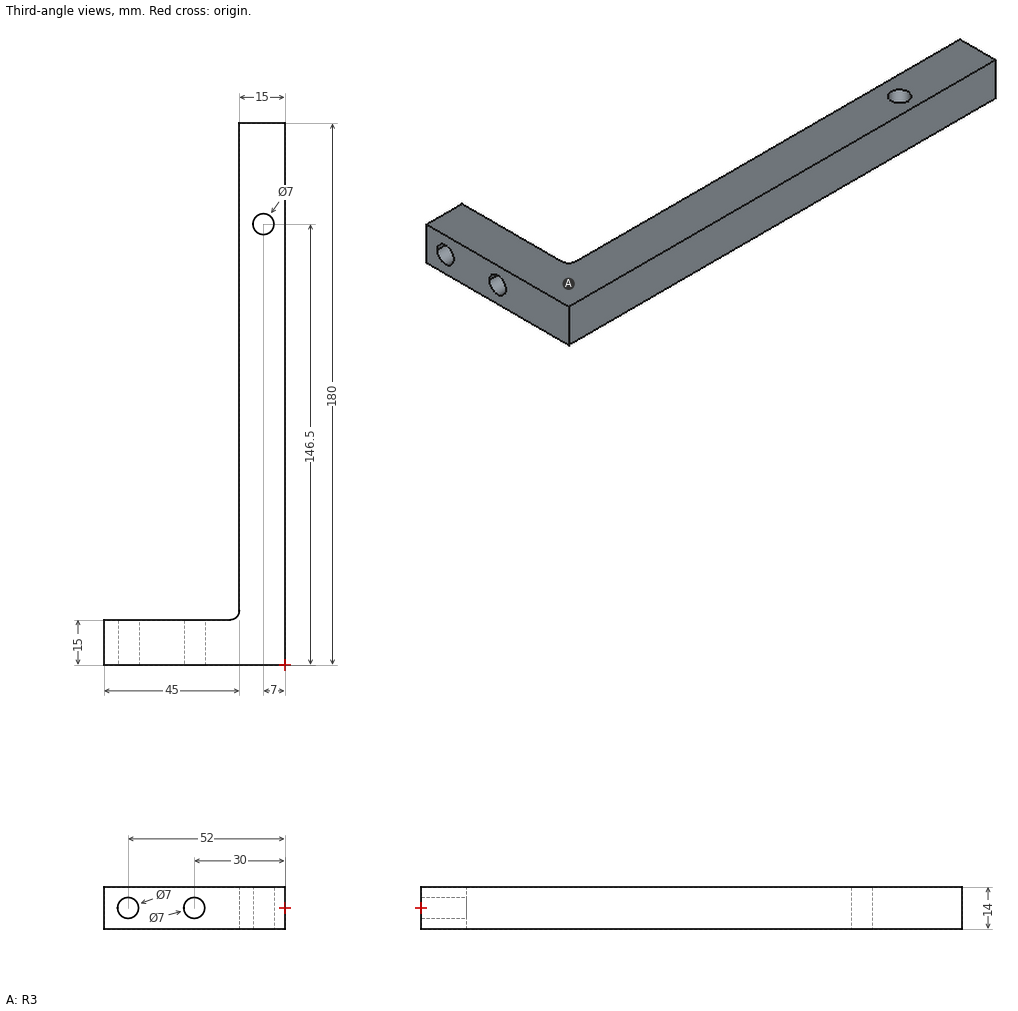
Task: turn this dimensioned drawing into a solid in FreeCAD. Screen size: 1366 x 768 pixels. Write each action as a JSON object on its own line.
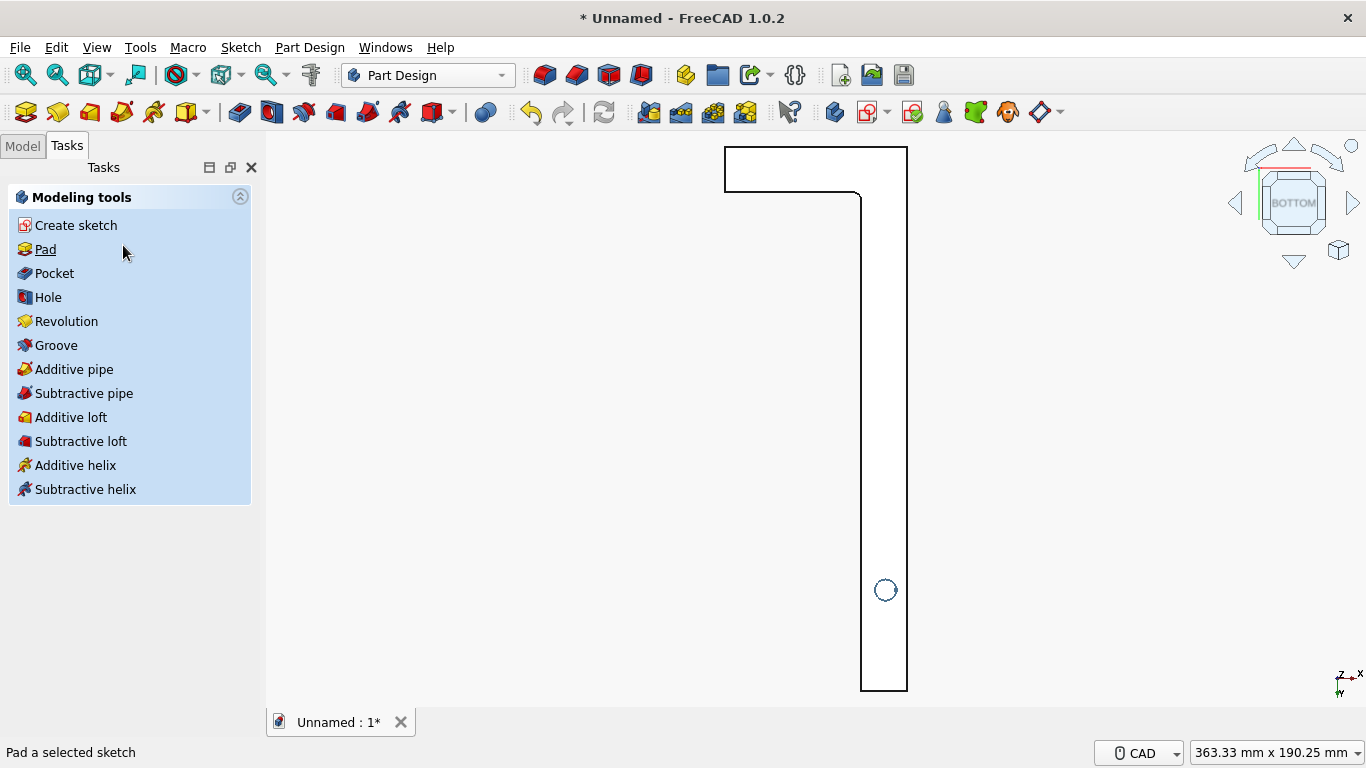
{"action": "left_click", "coordinate": [240, 112]}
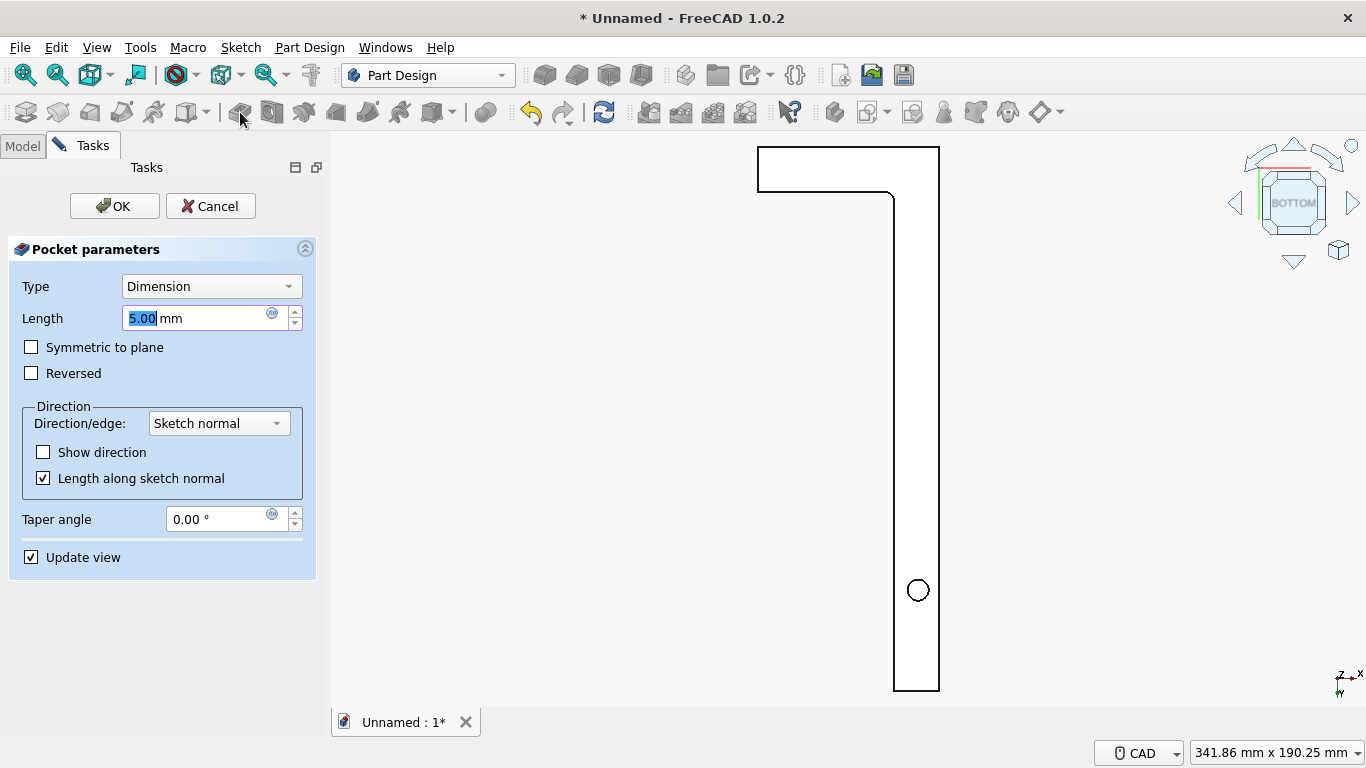
{"action": "left_click", "coordinate": [212, 286]}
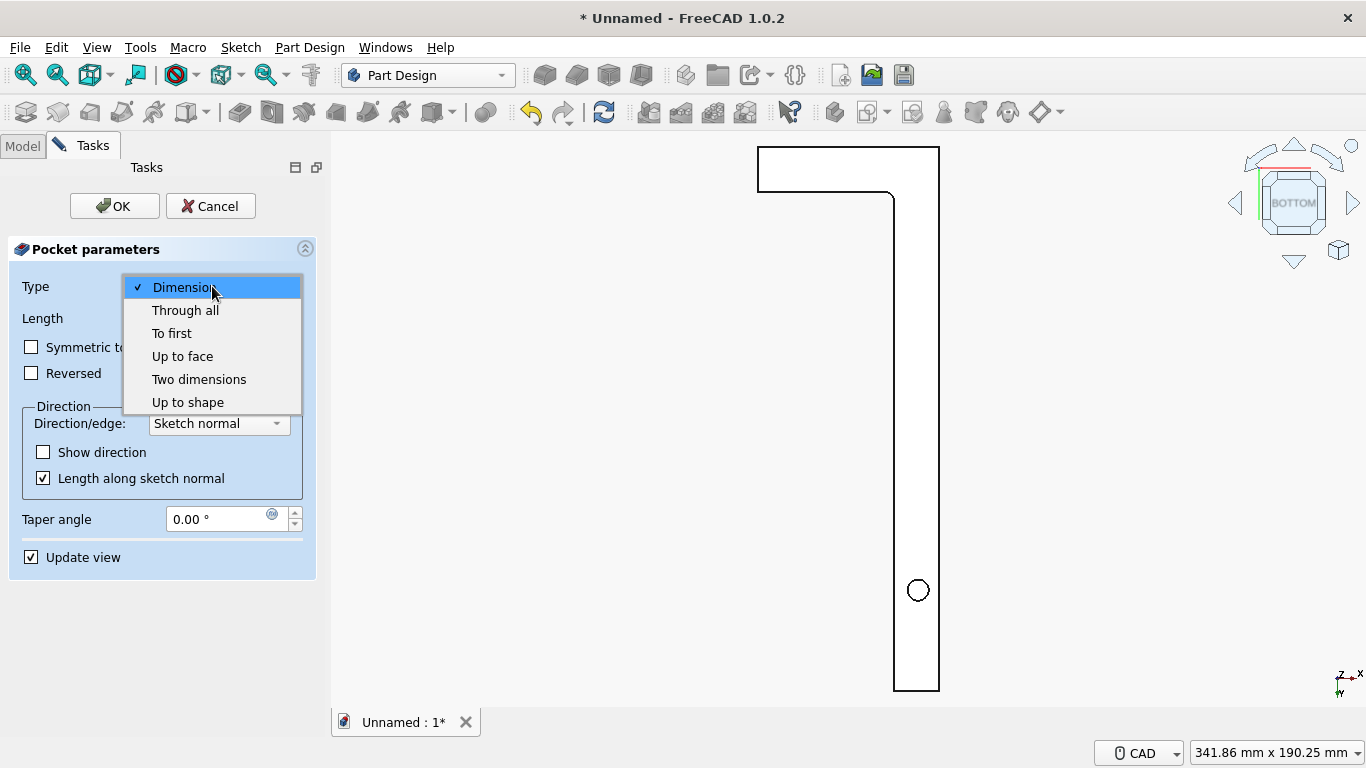
{"action": "left_click", "coordinate": [212, 334]}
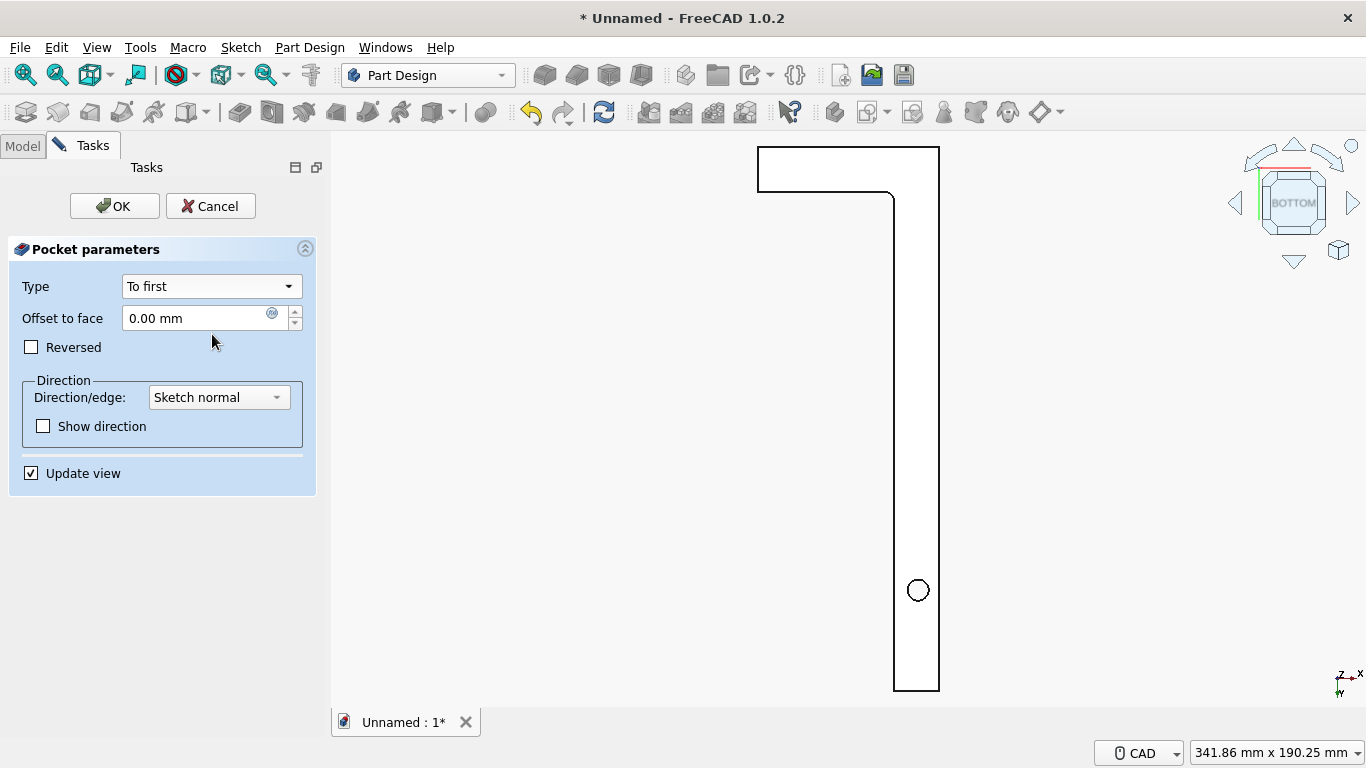
{"action": "left_click", "coordinate": [115, 206]}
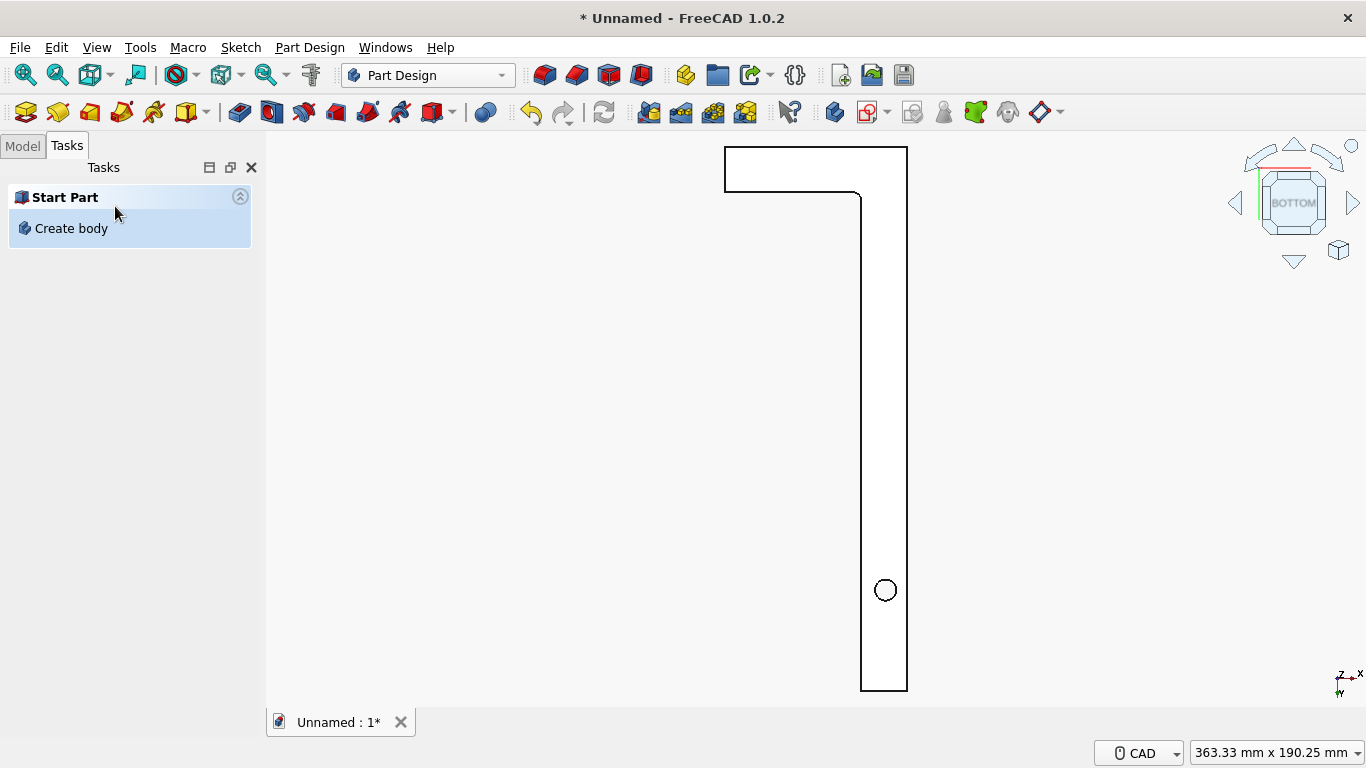
{"action": "key", "text": "0"}